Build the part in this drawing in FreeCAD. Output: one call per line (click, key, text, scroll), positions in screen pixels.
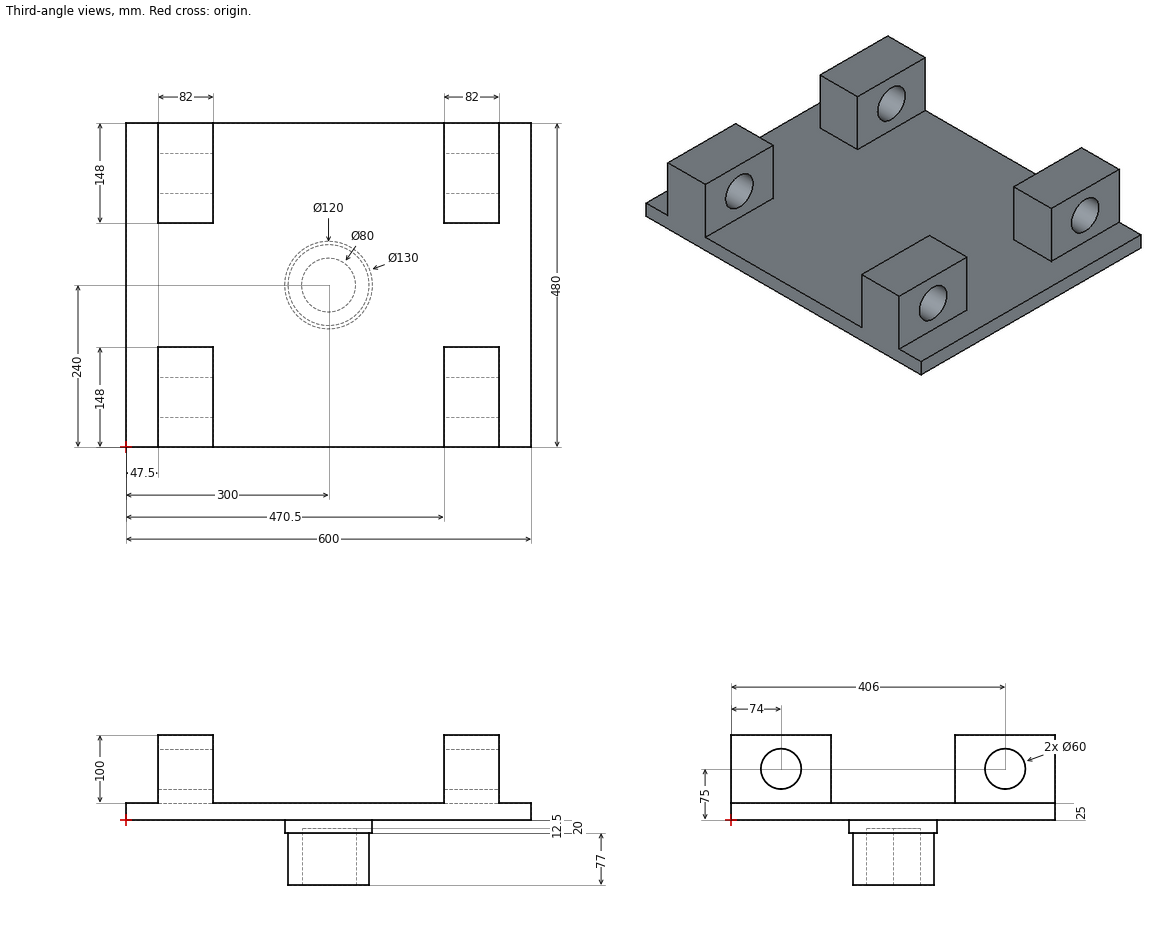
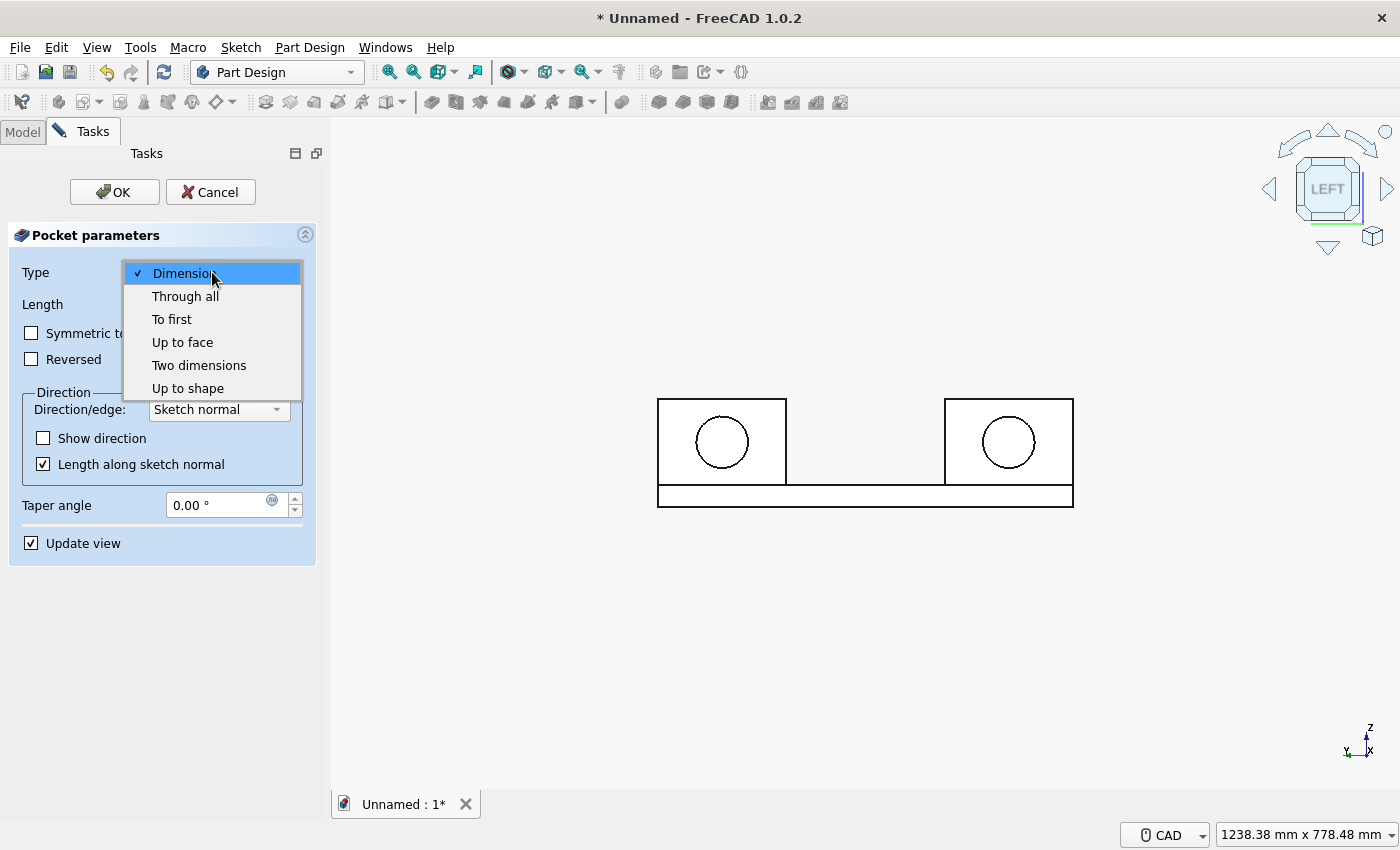
click(212, 296)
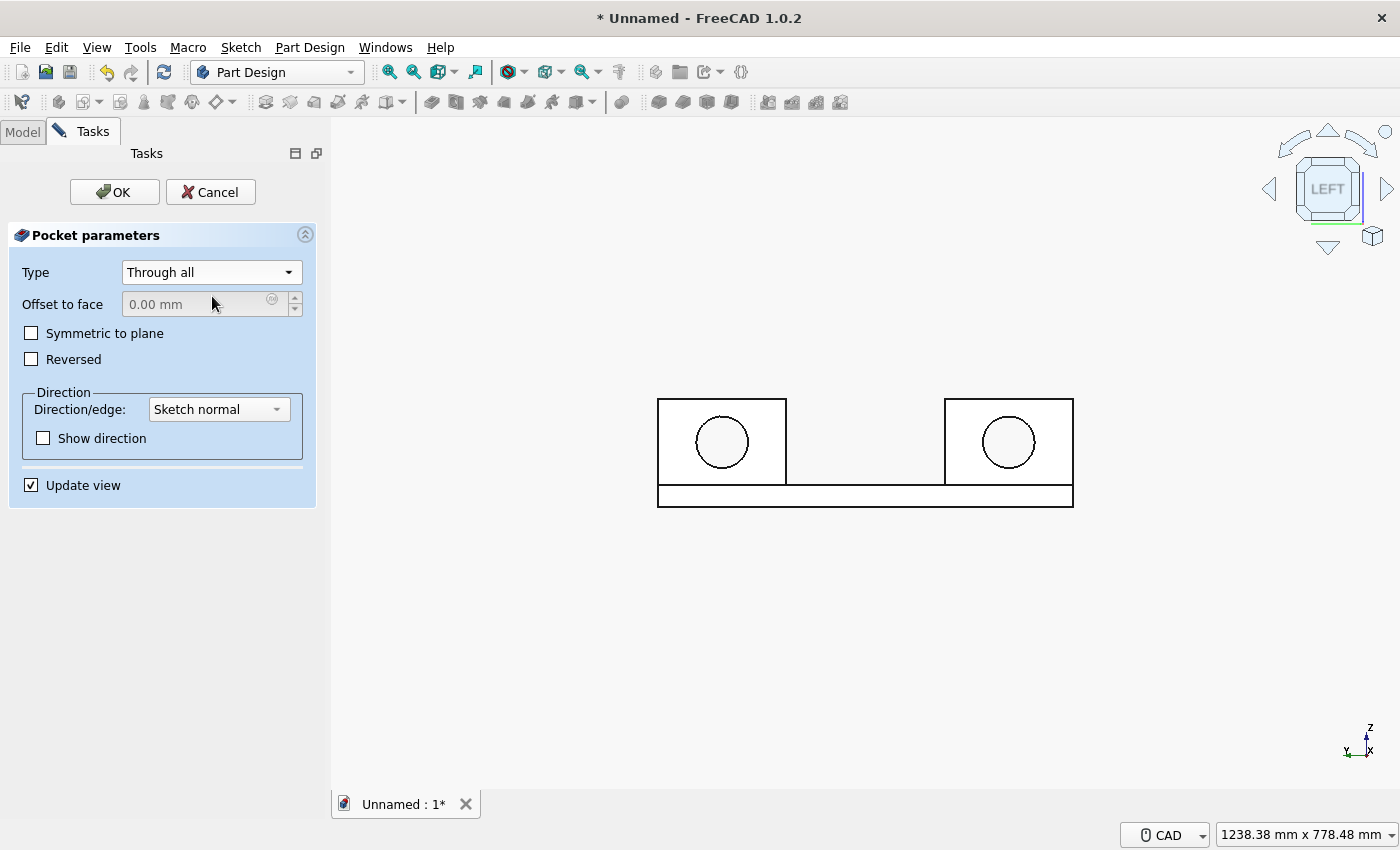
click(115, 192)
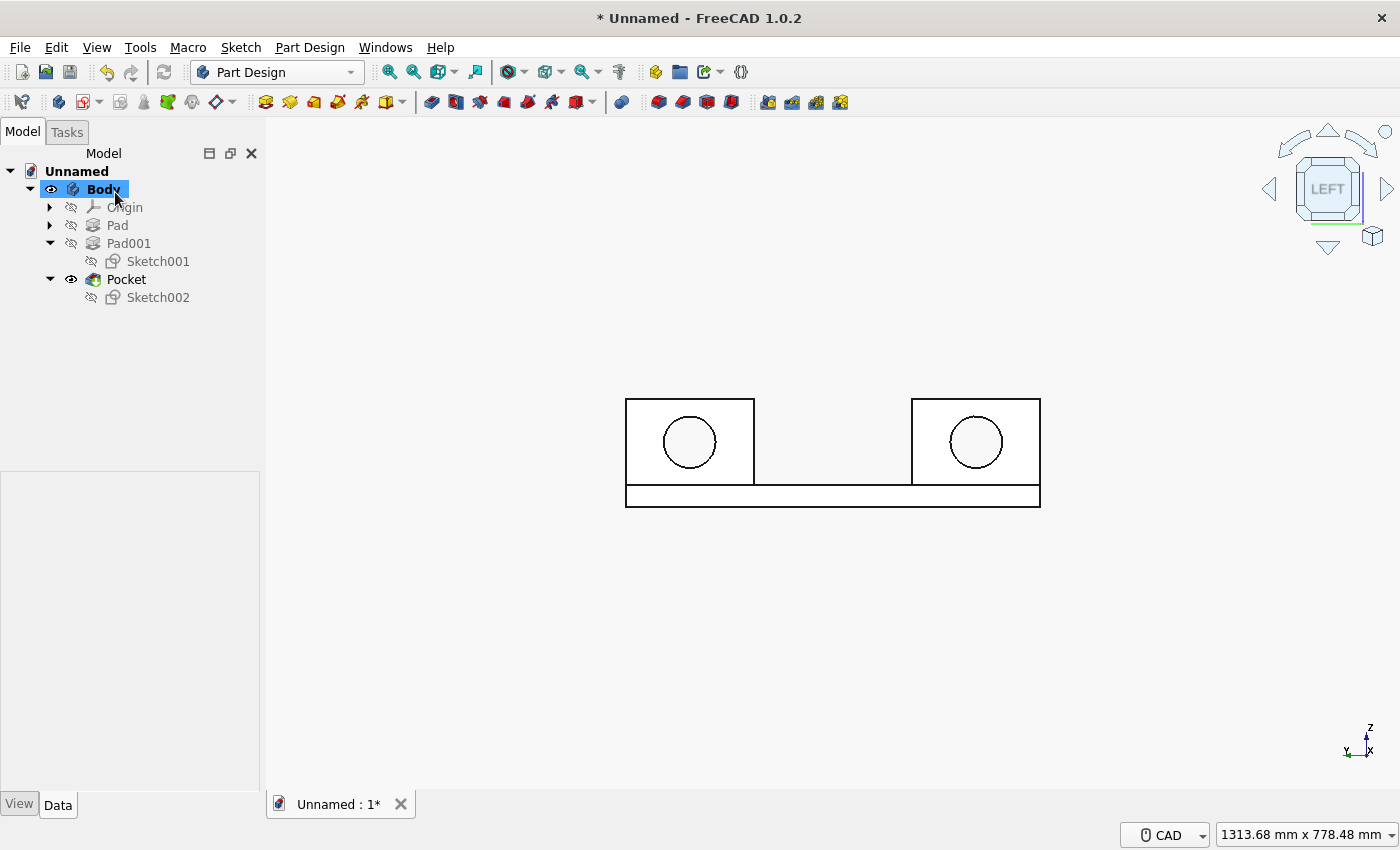
click(390, 72)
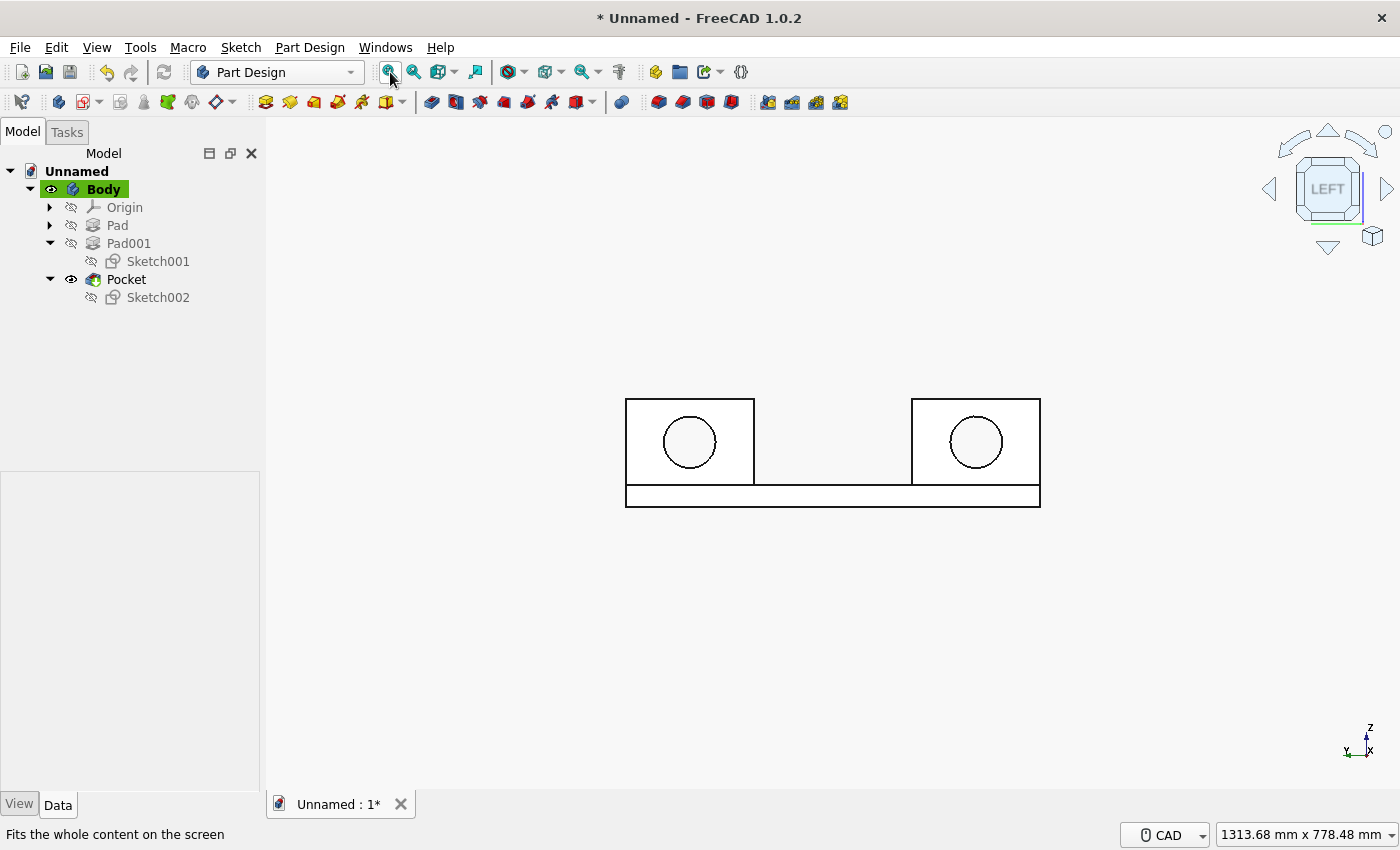
click(84, 102)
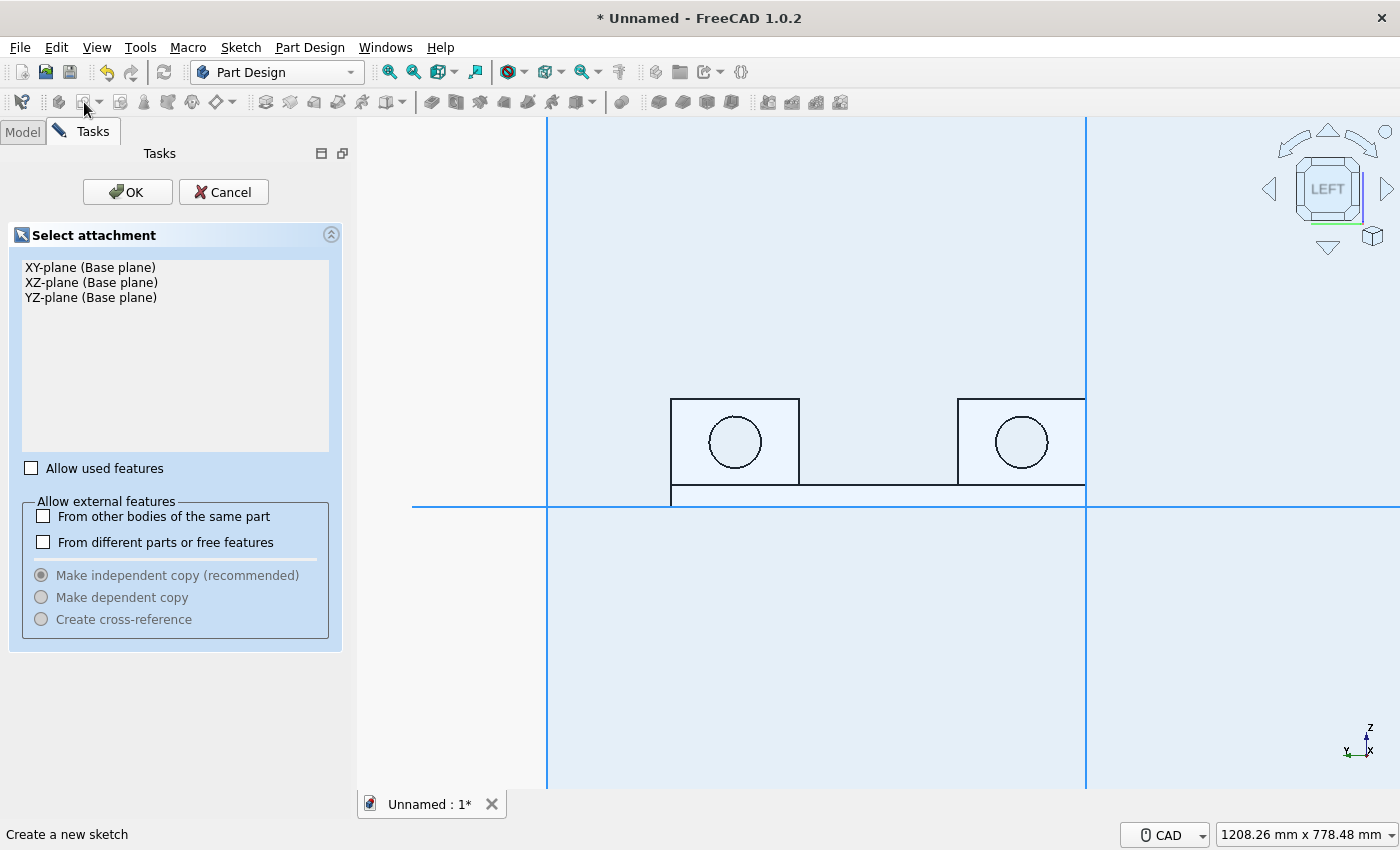
click(82, 268)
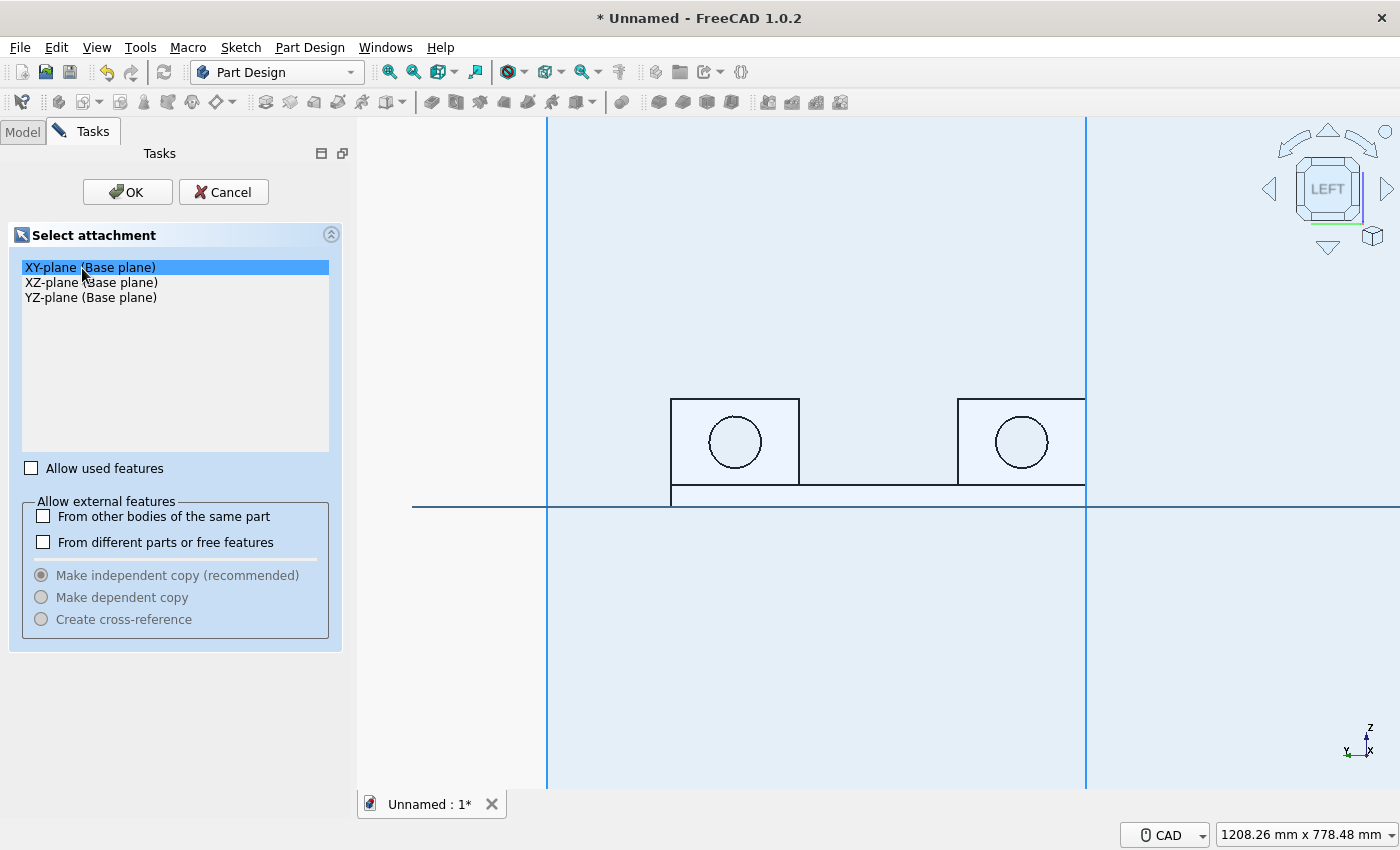
click(128, 192)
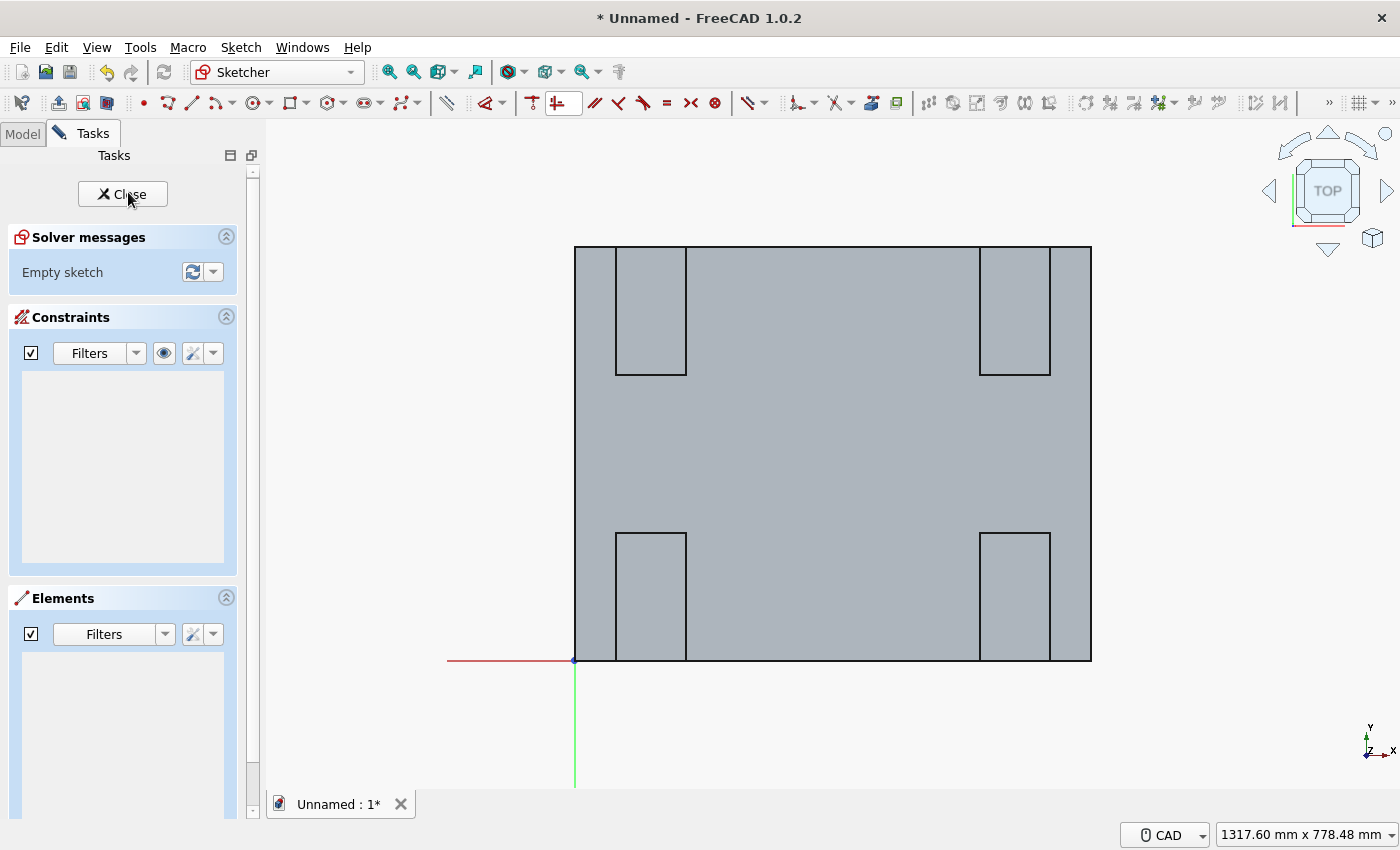
click(108, 104)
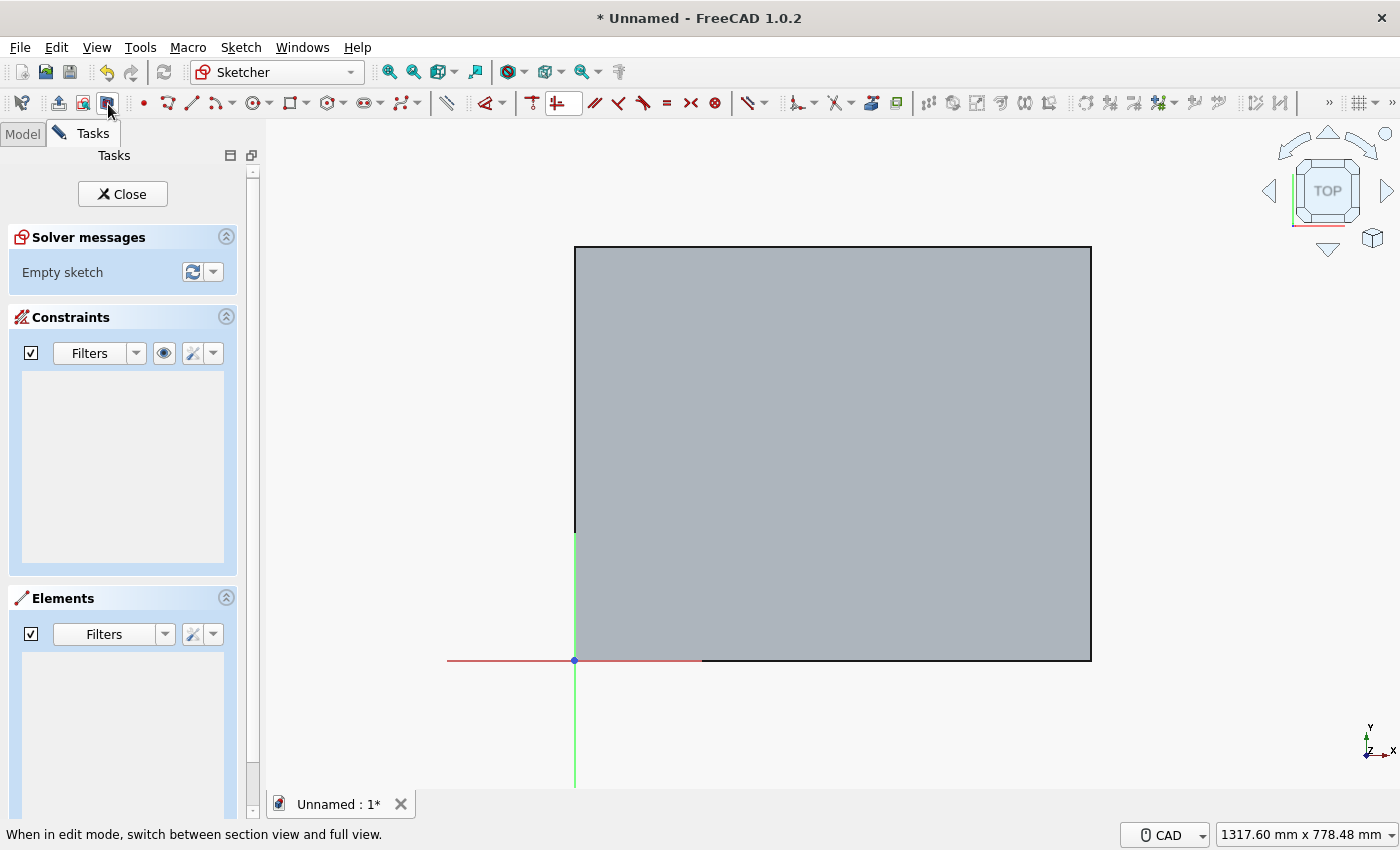
scroll(855, 454, up, 7)